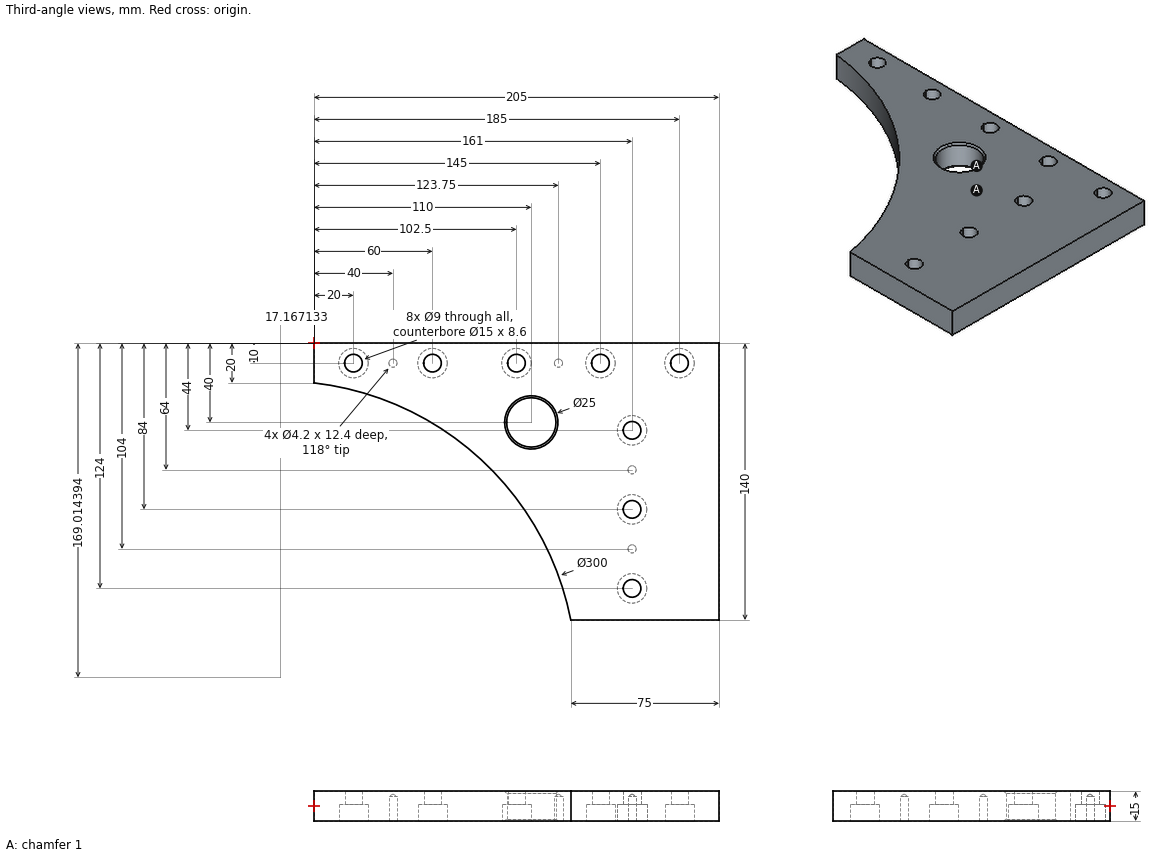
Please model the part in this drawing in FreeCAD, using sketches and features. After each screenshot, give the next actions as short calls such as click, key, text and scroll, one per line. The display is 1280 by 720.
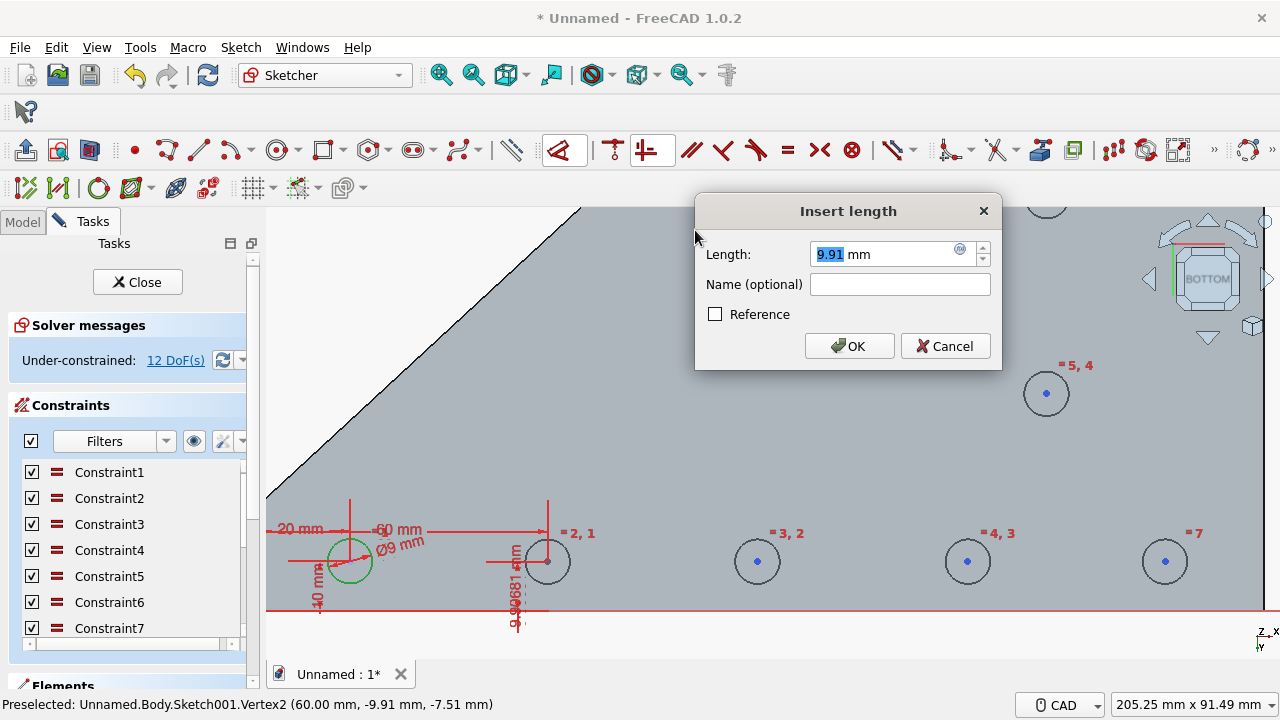
text(10)
key(Return)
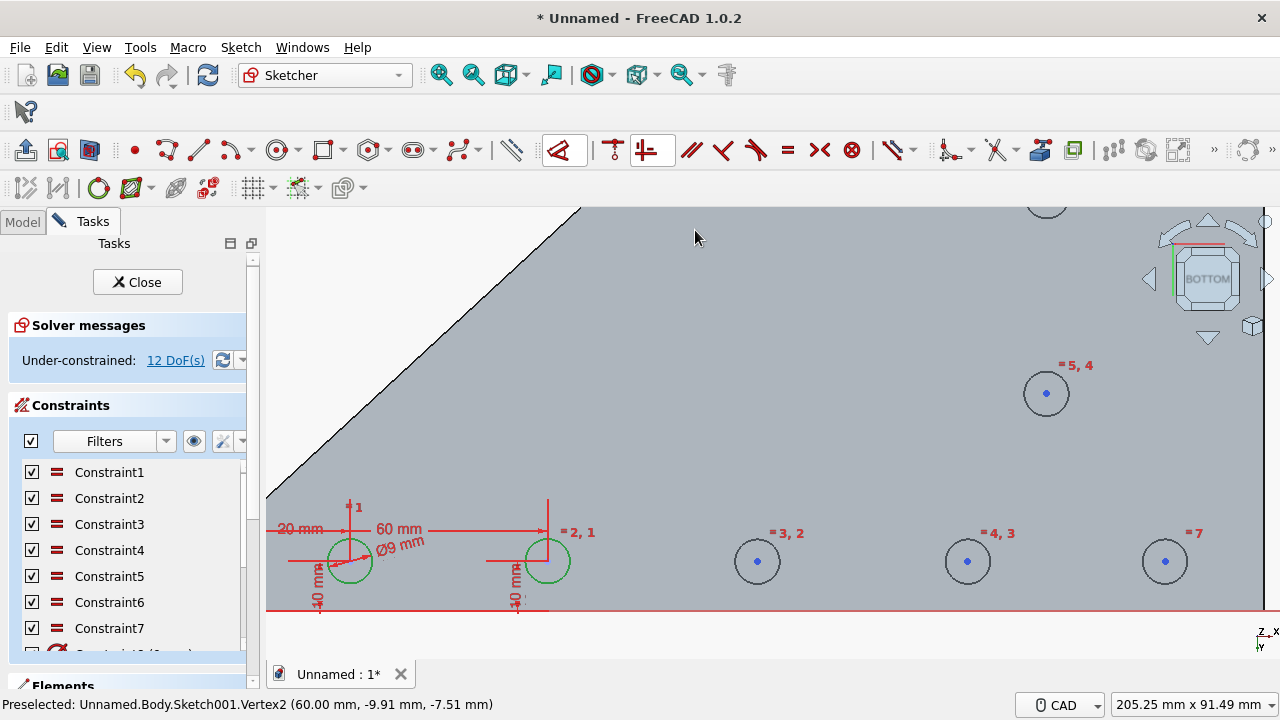
click(757, 562)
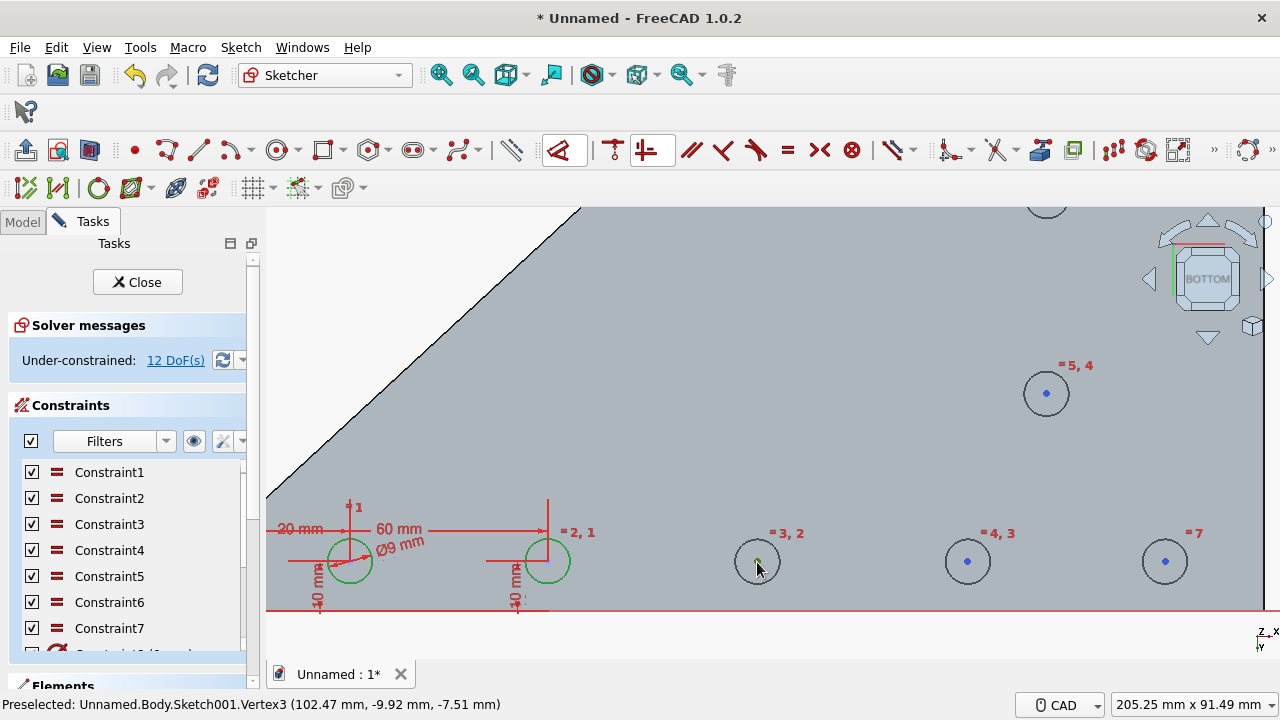
click(582, 150)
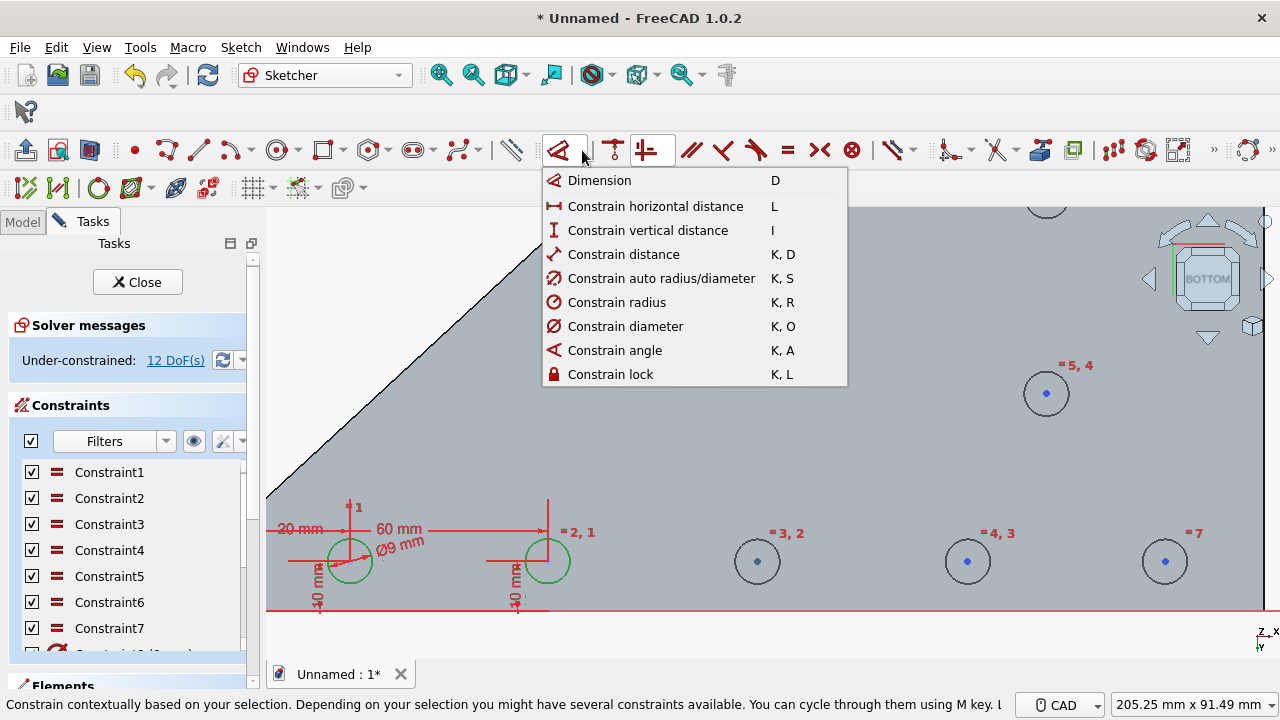
click(695, 230)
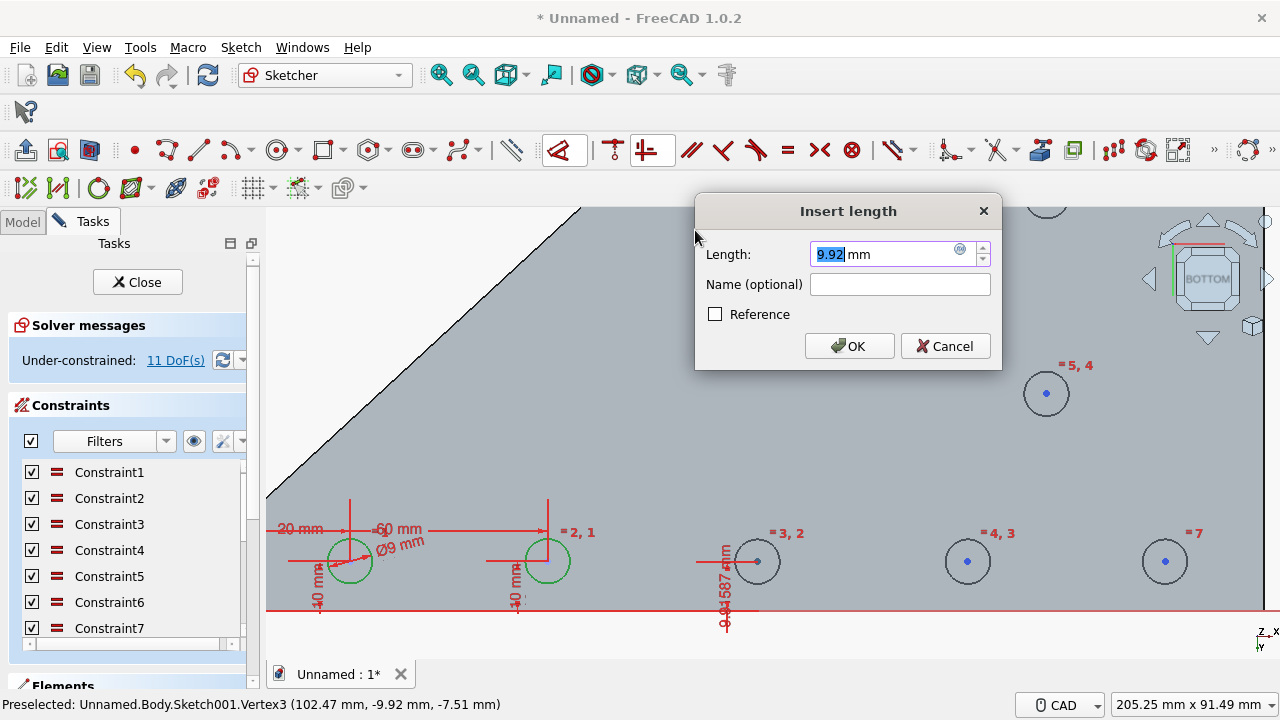
text(10)
key(Return)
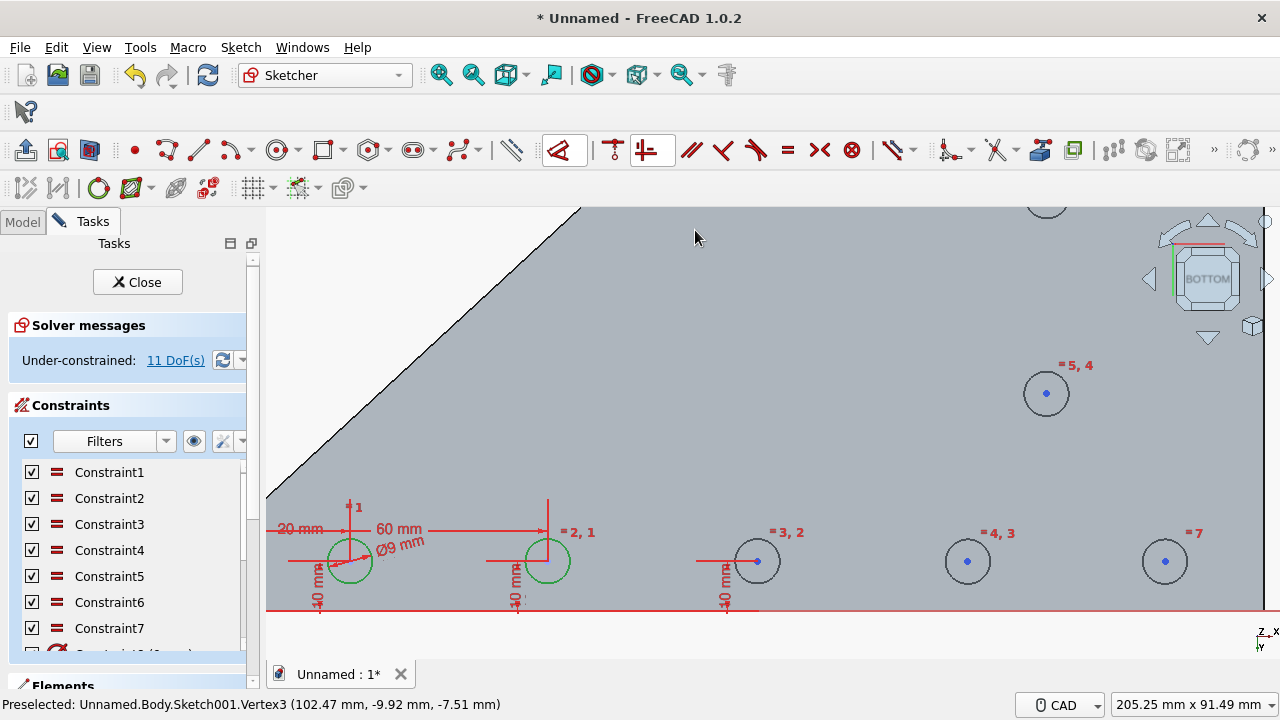
click(968, 562)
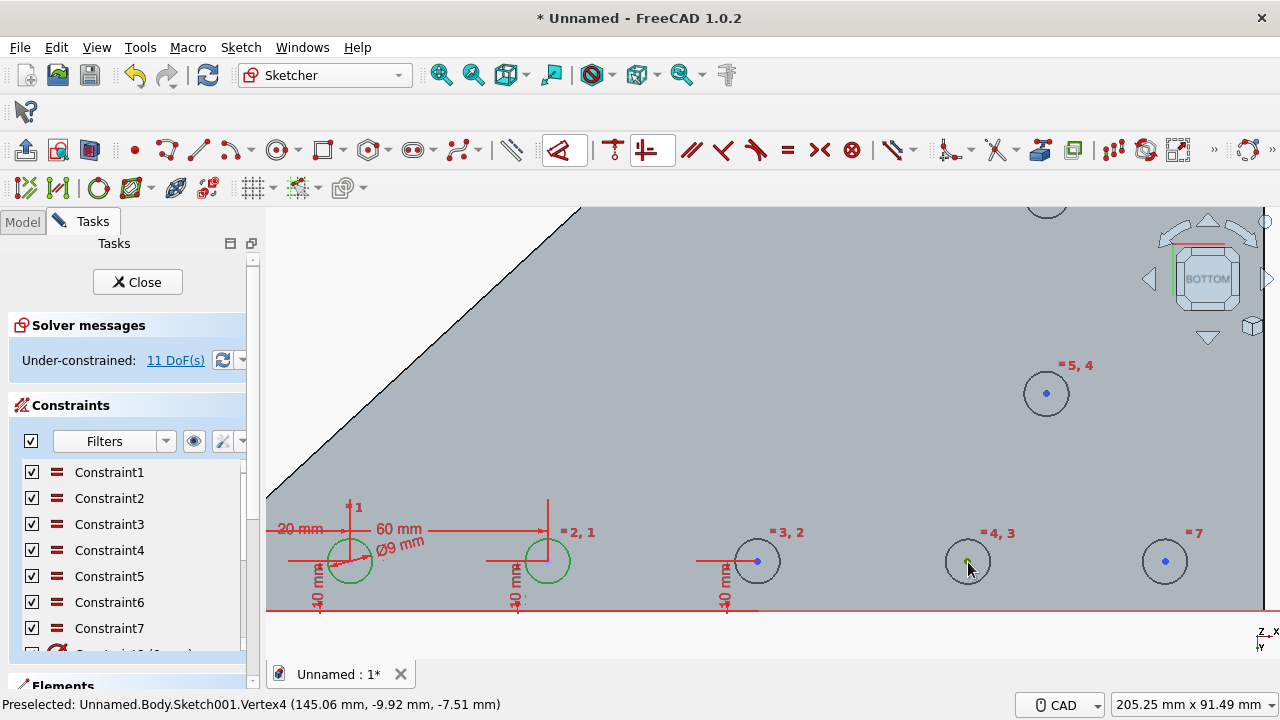
key(i)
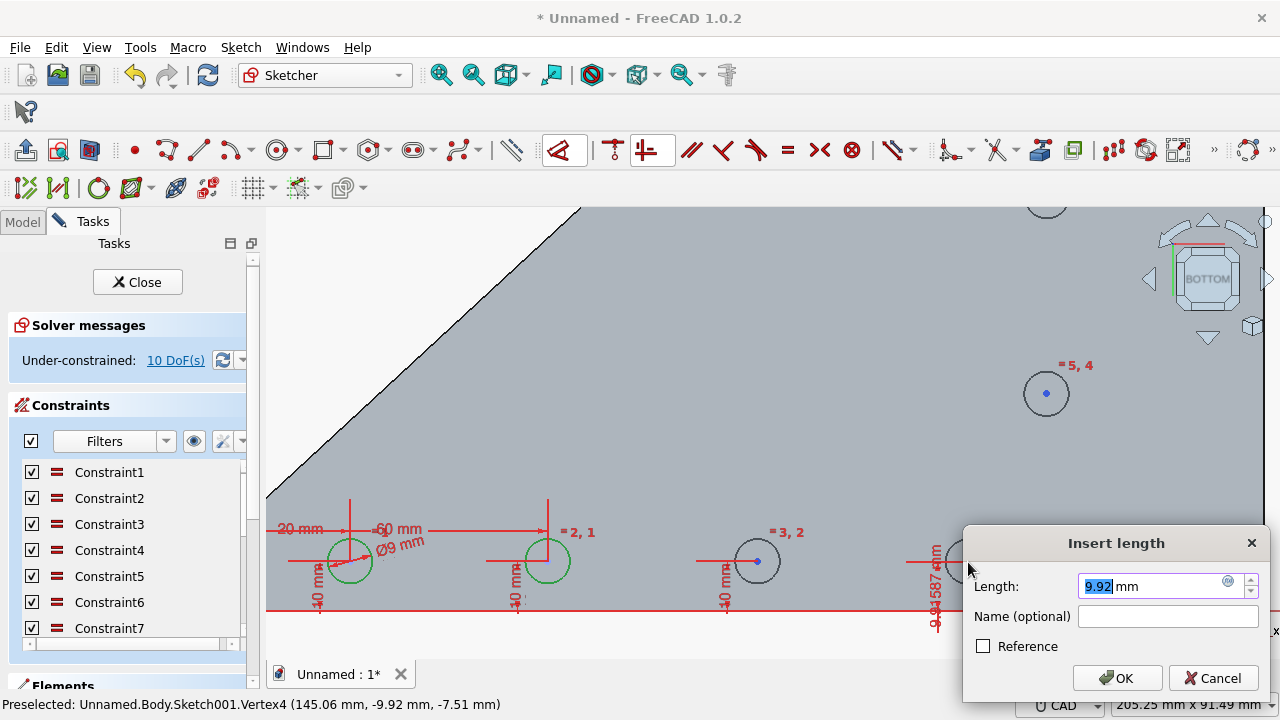
text(10)
key(Return)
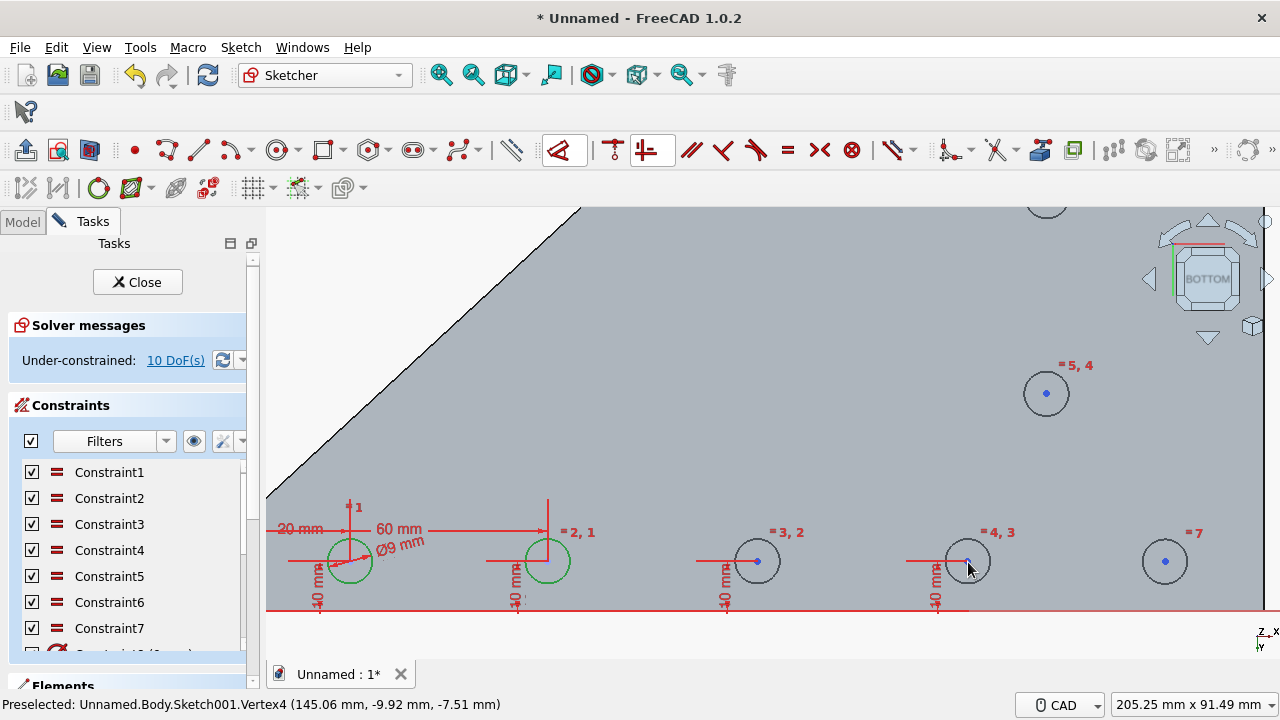
click(1046, 394)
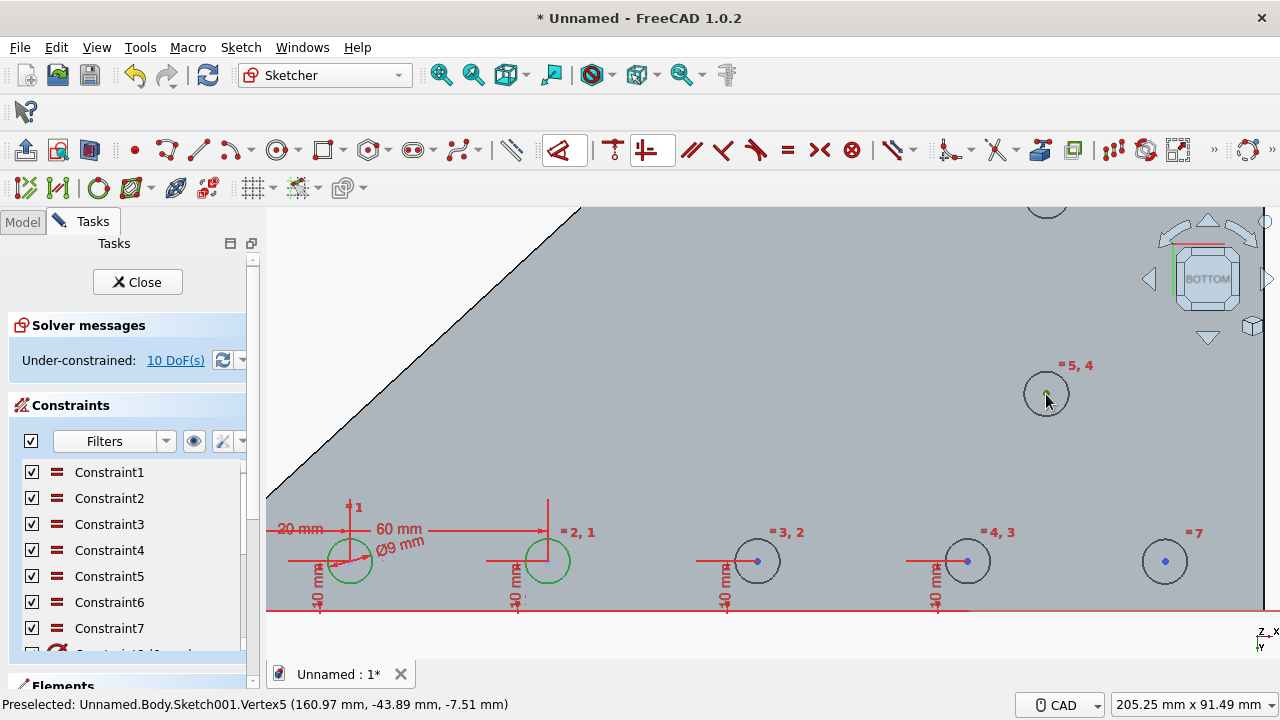
key(i)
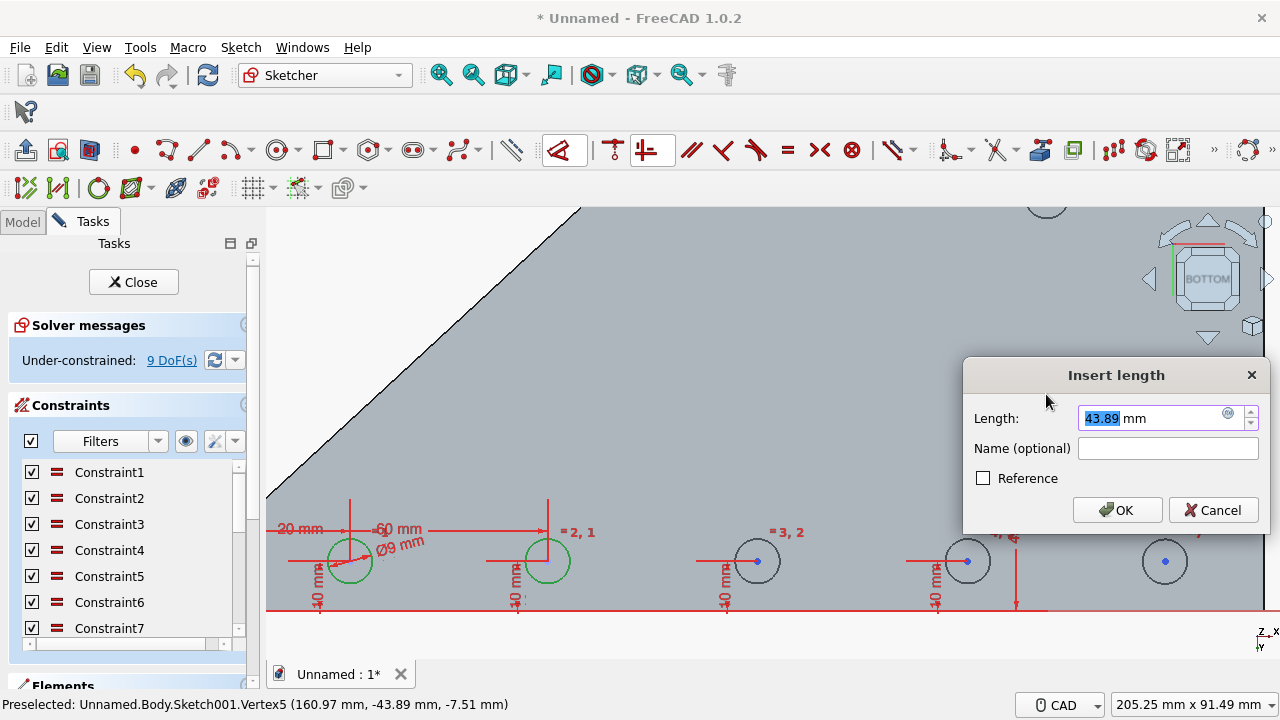
text(44)
key(Return)